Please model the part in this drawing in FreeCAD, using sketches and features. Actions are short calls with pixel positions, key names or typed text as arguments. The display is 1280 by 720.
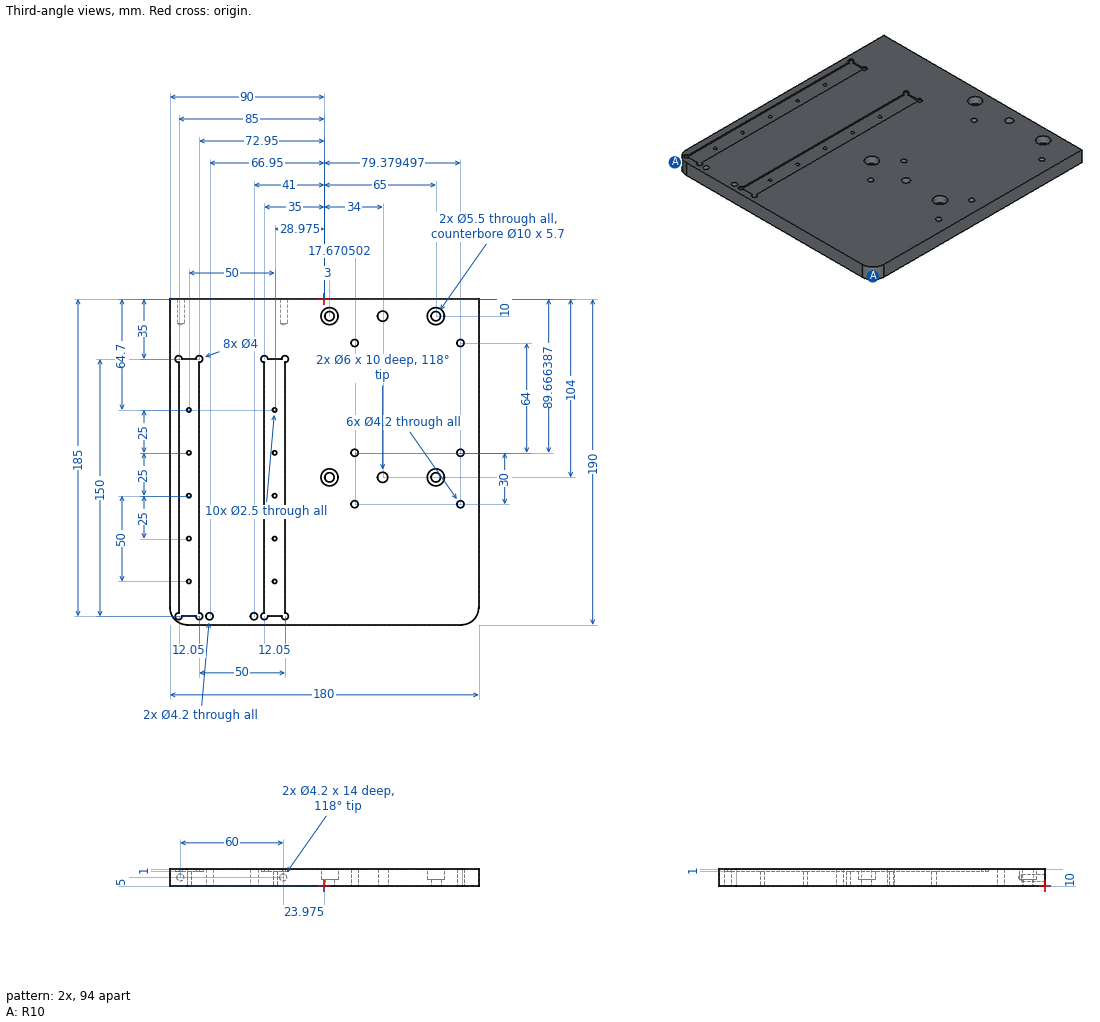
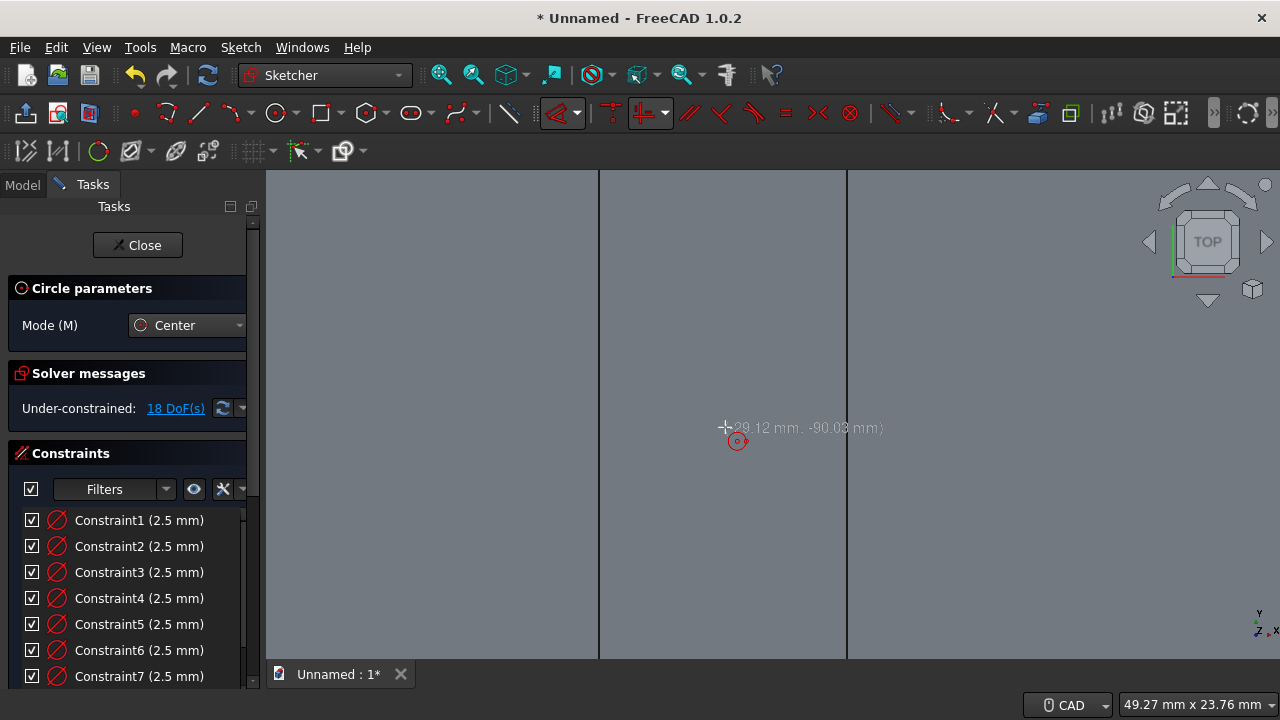
scroll(725, 427, down, 12)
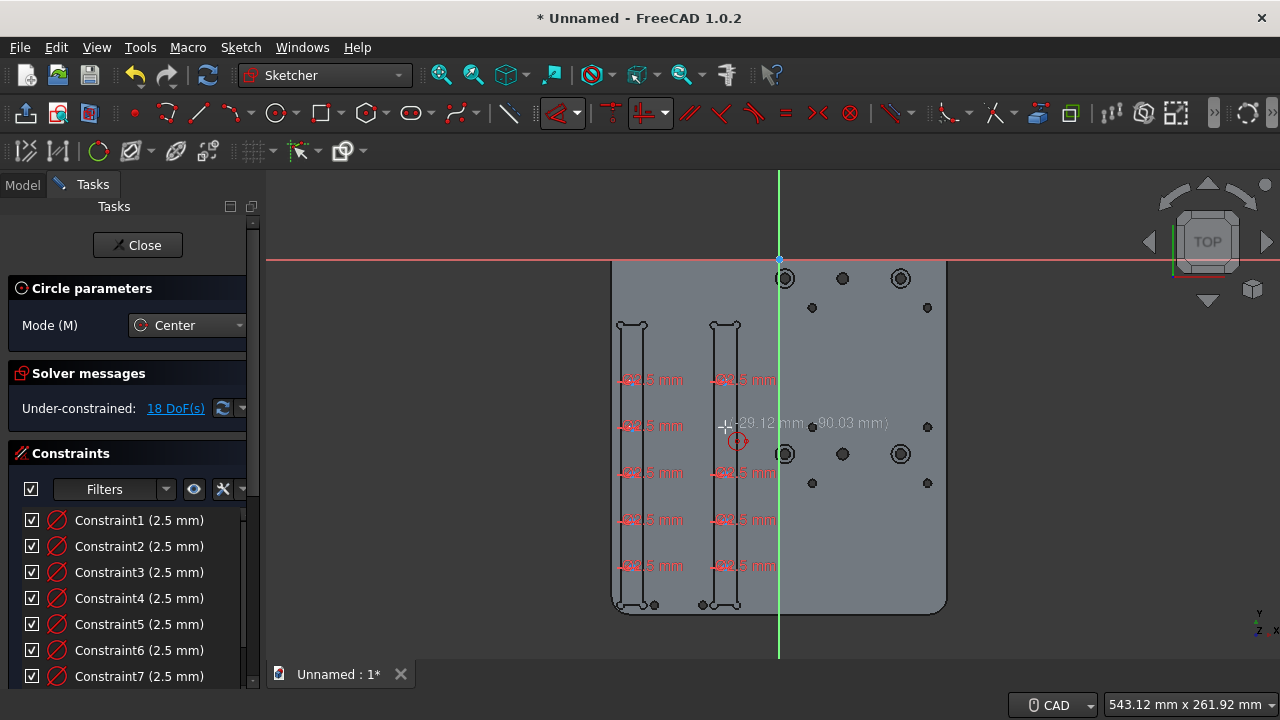
click(725, 427)
move(727, 426)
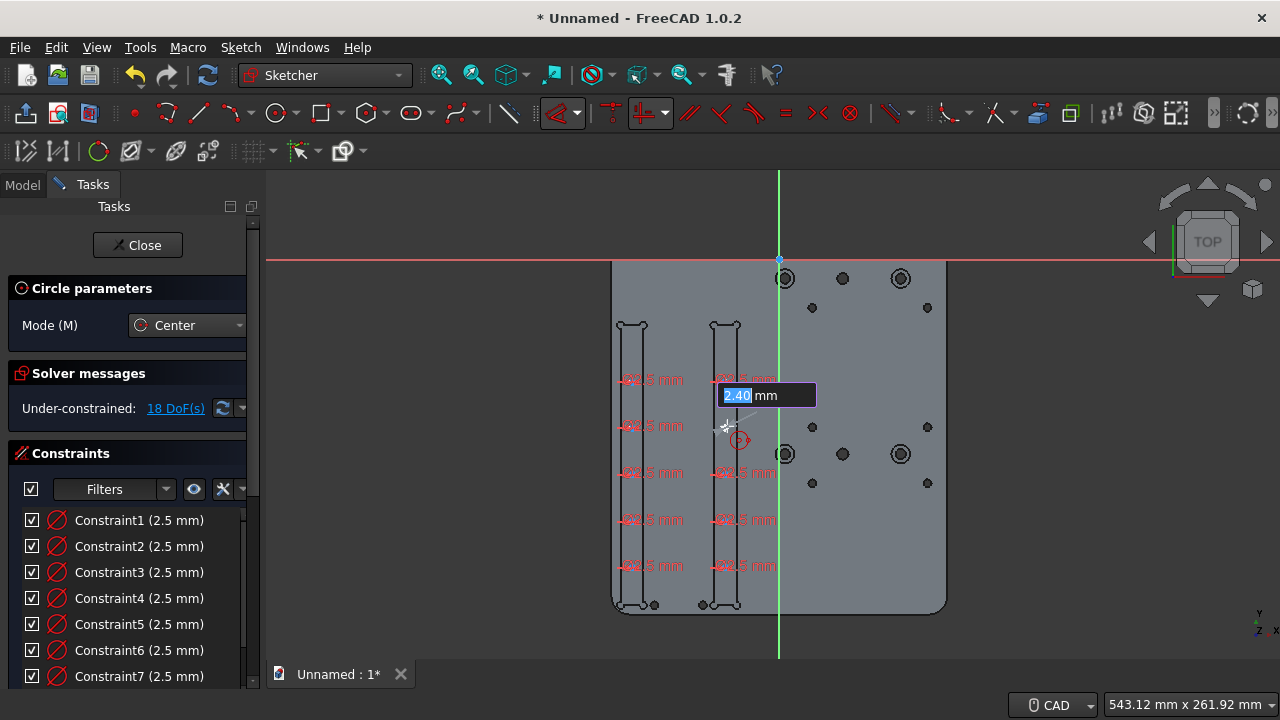
text(2.5)
key(Return)
key(Escape)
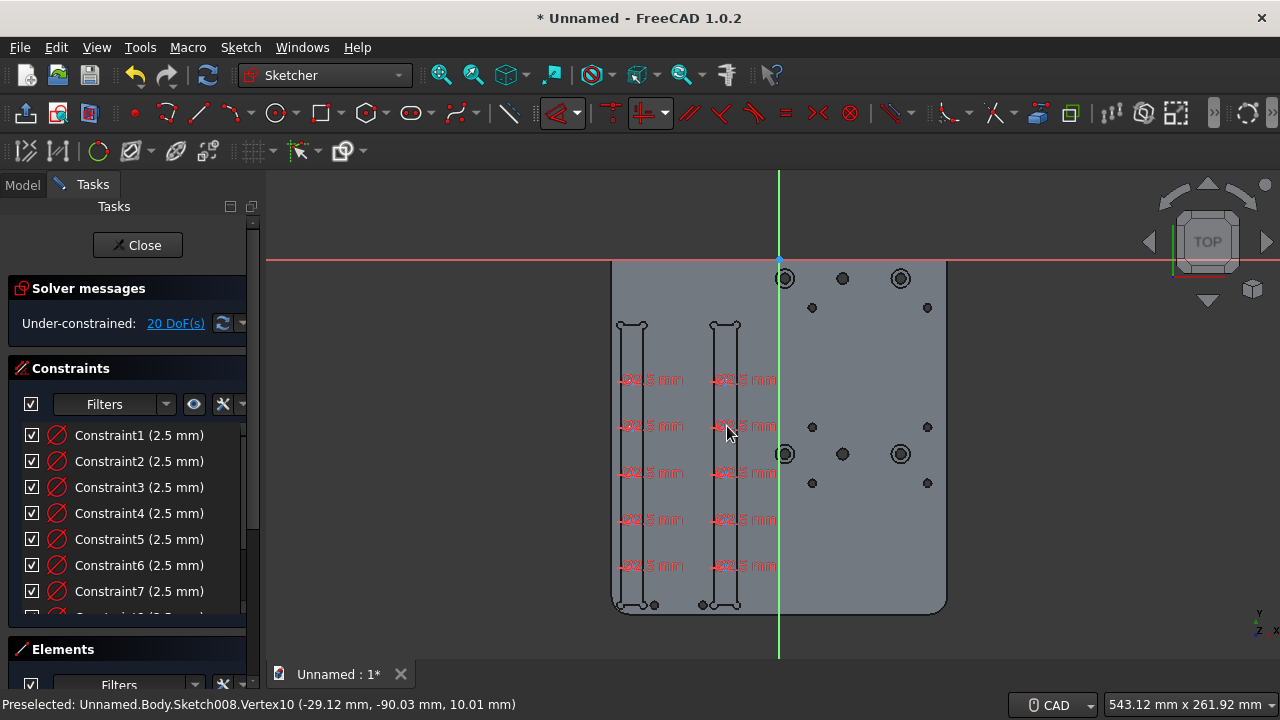
click(725, 382)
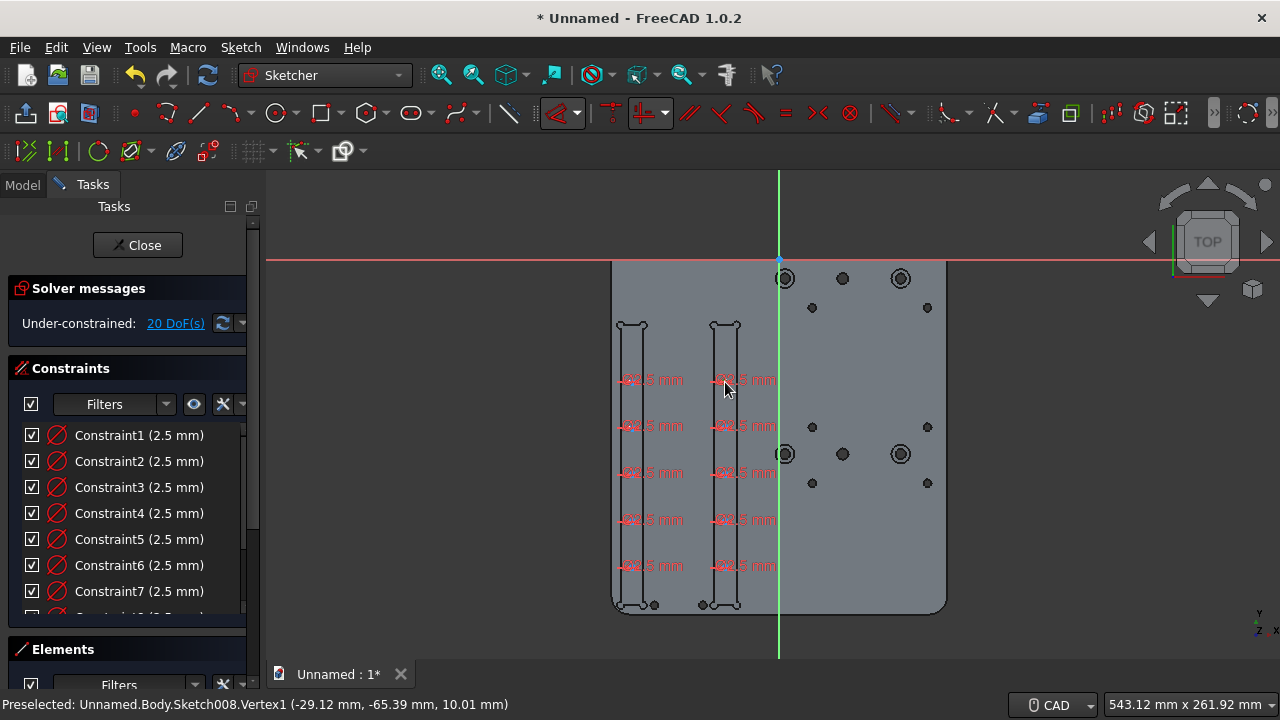
click(632, 382)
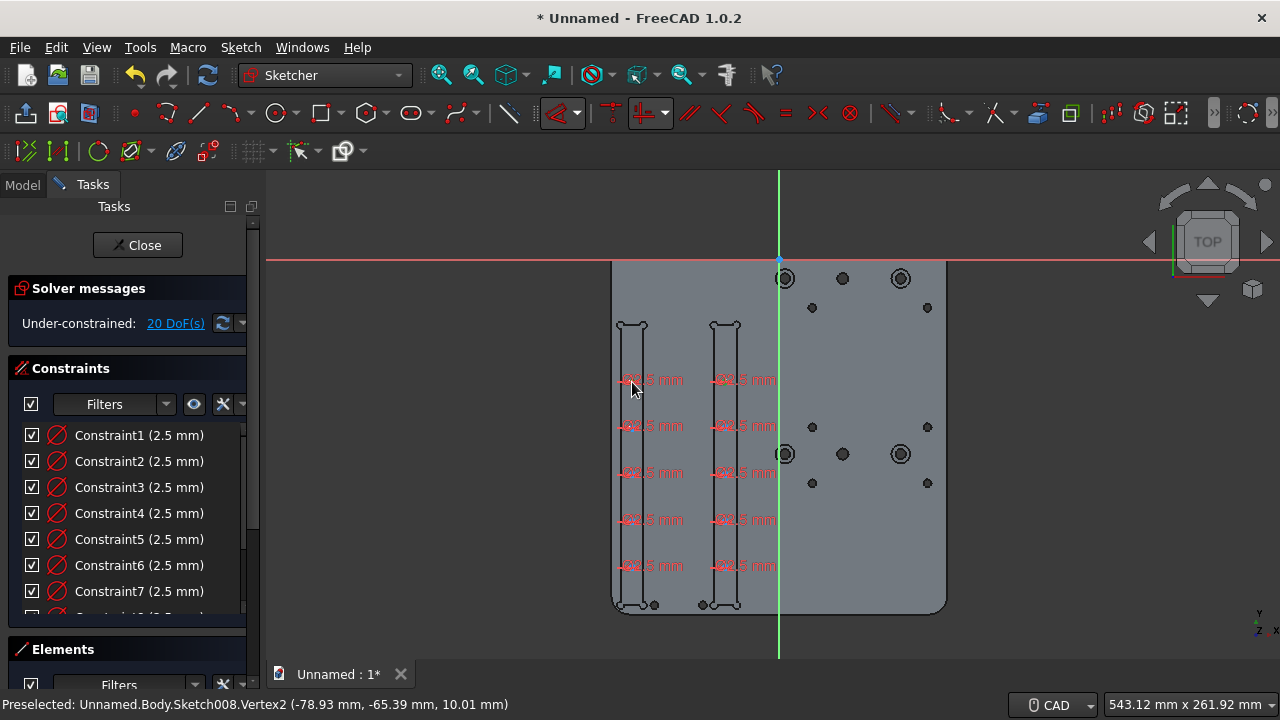
key(h)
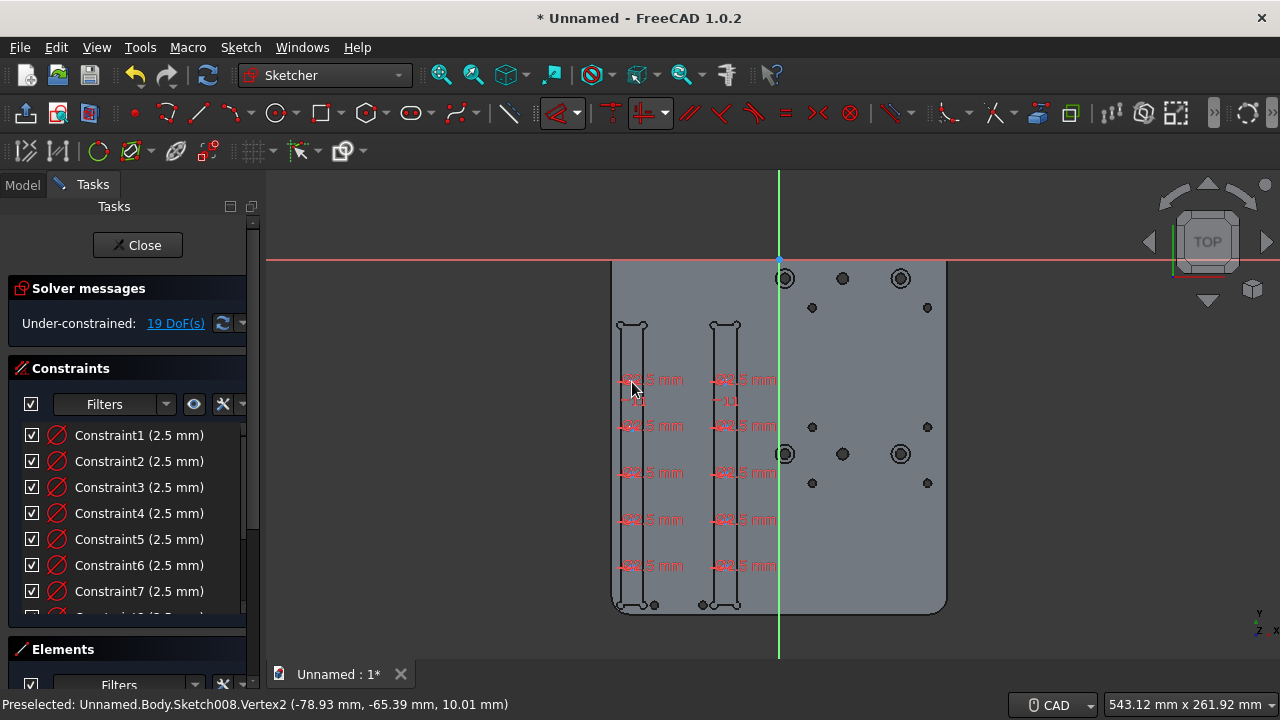
click(632, 382)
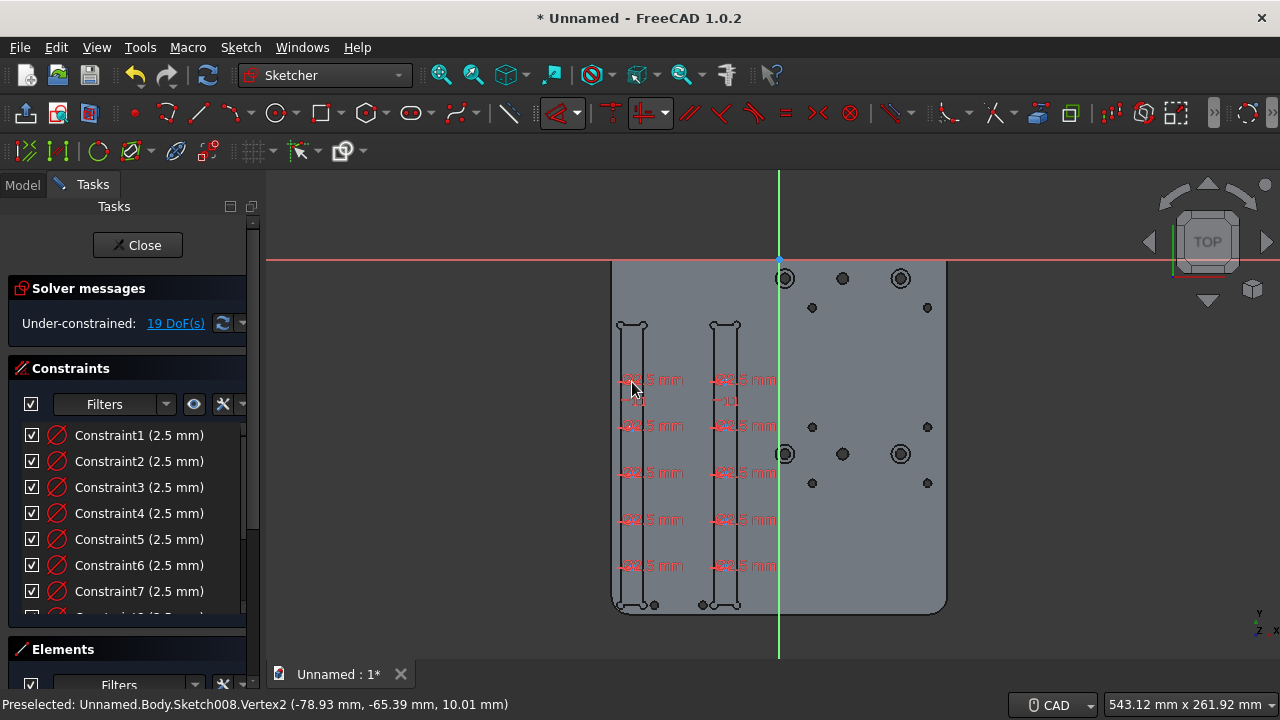
click(632, 428)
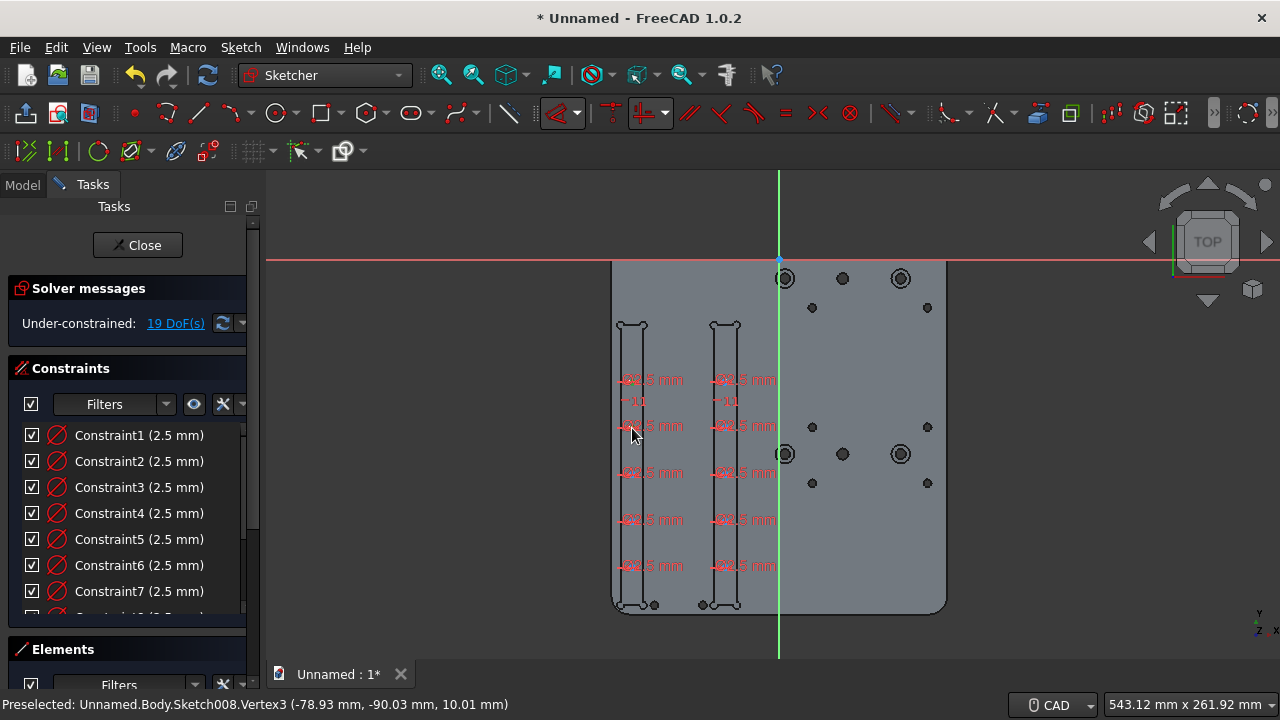
key(v)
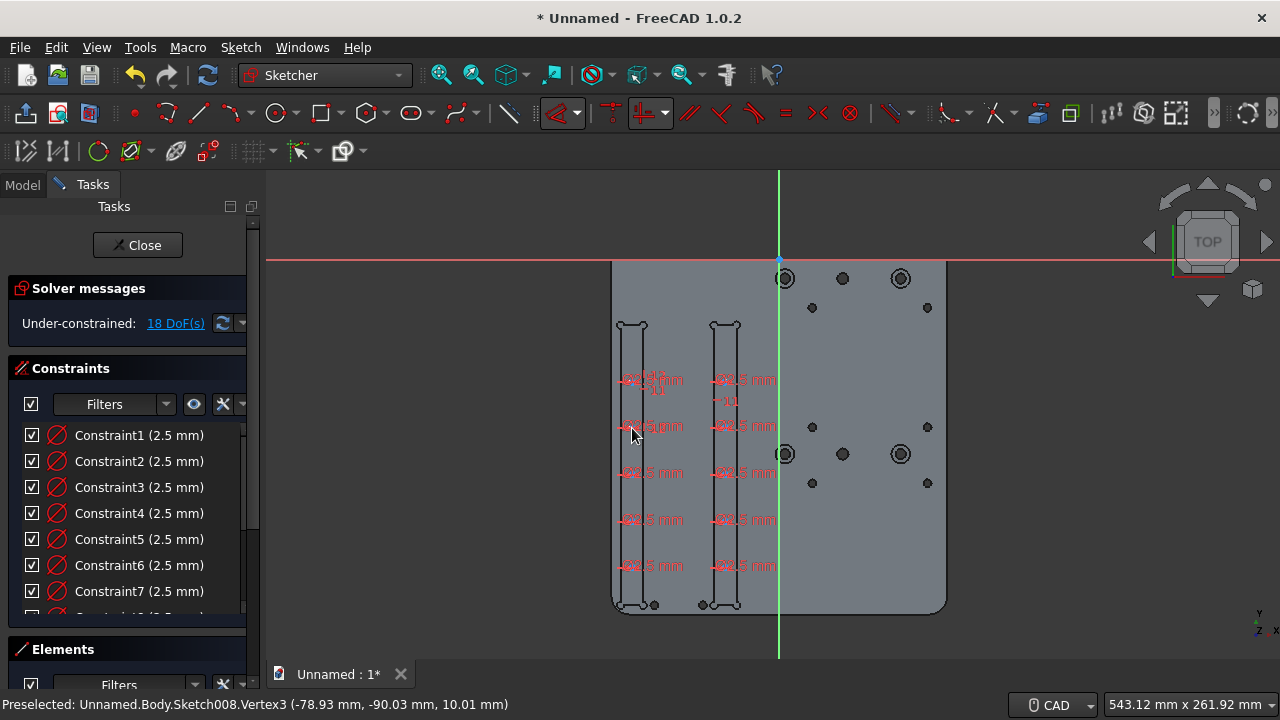
click(632, 428)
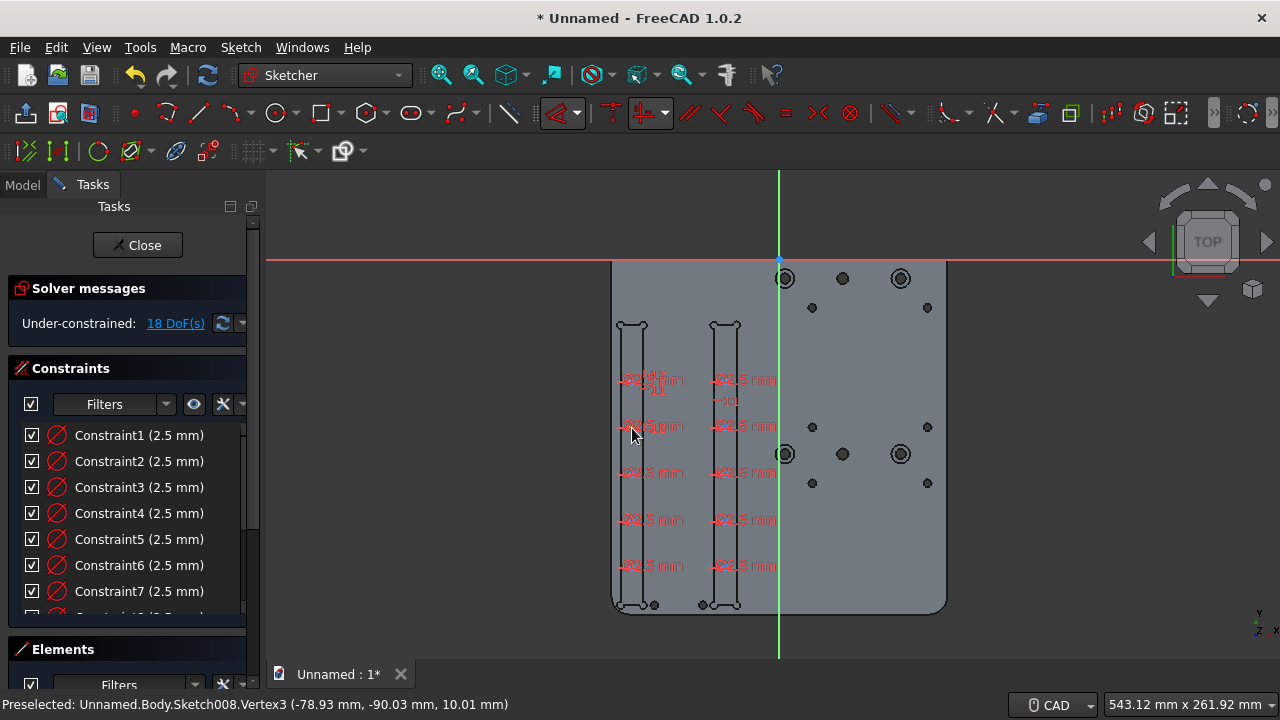
click(632, 475)